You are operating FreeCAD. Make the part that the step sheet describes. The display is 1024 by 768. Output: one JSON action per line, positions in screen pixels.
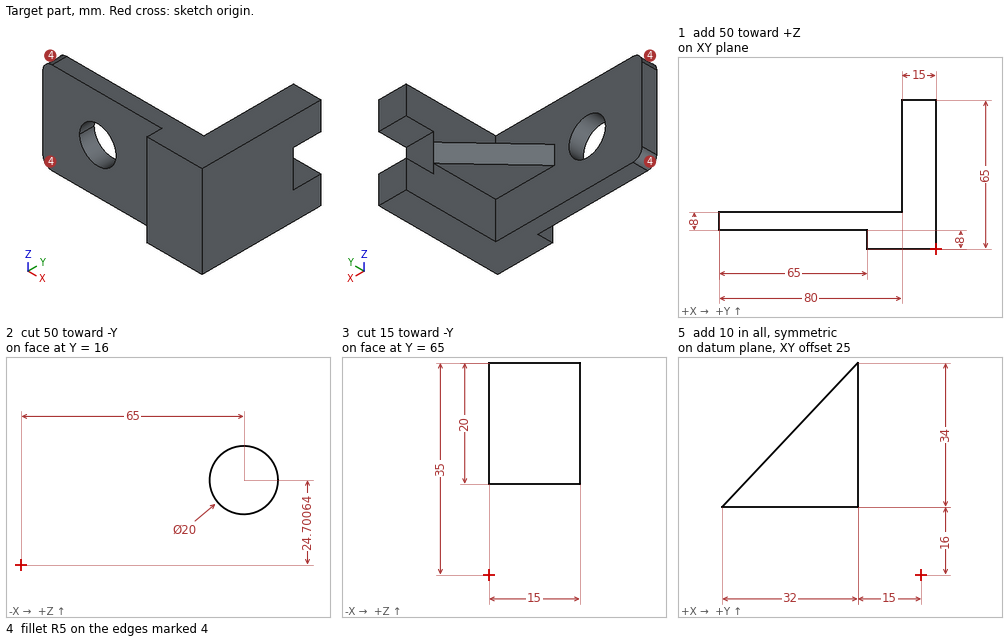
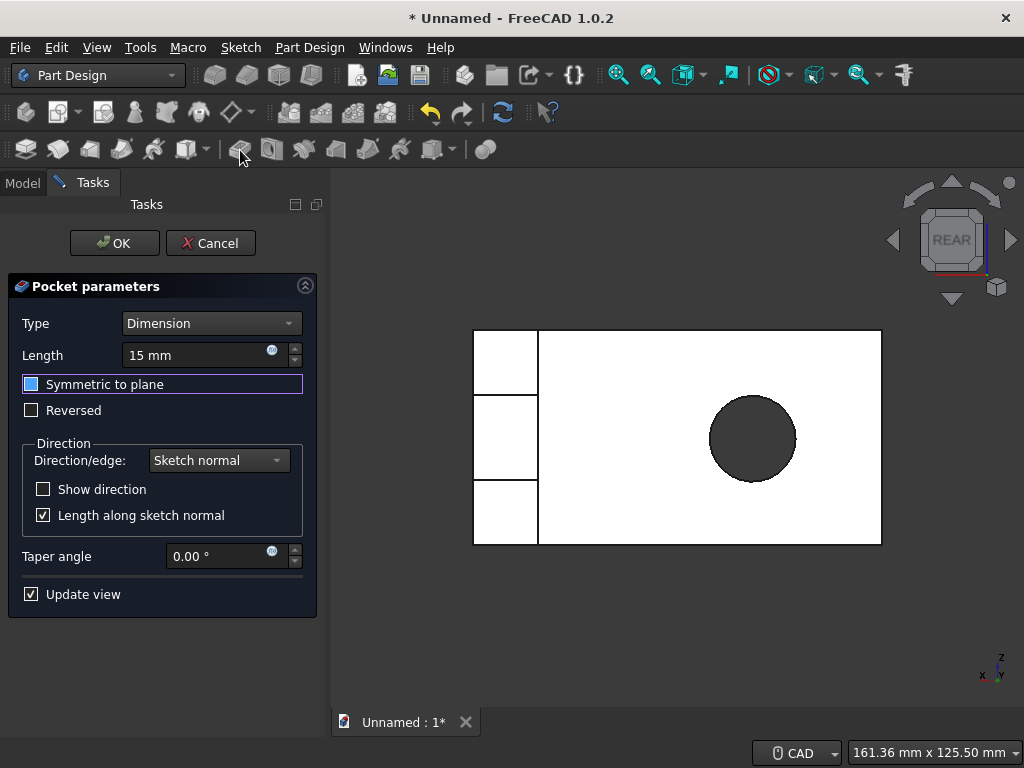
{"action": "left_click", "coordinate": [115, 243]}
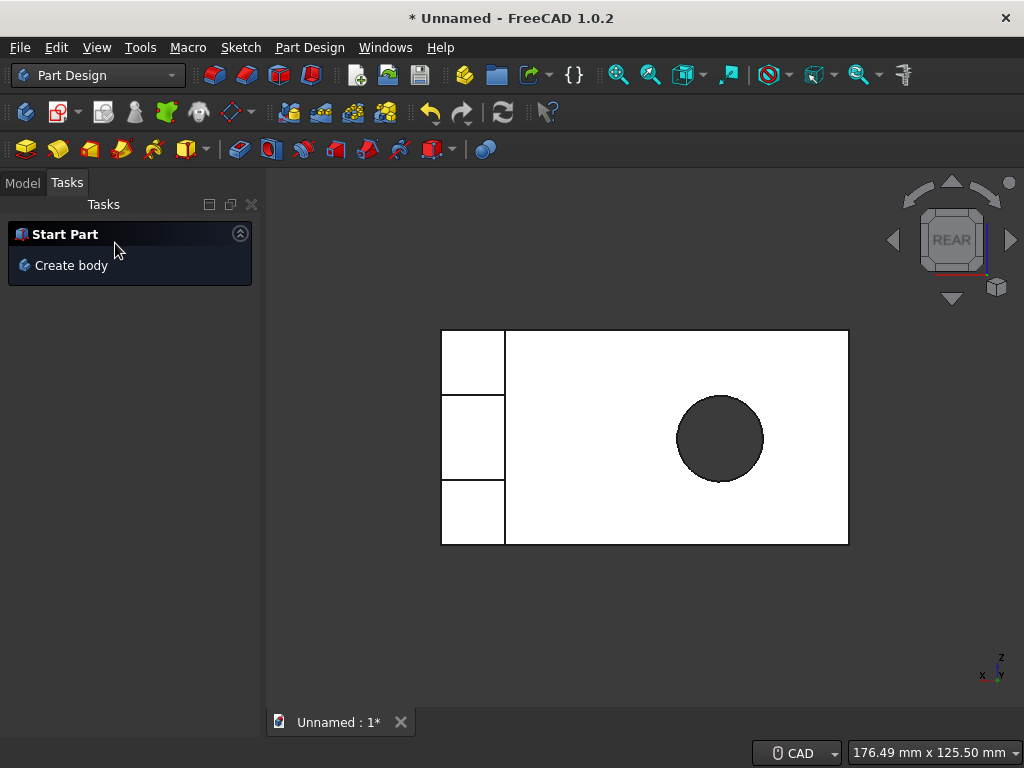
{"action": "key", "text": "0"}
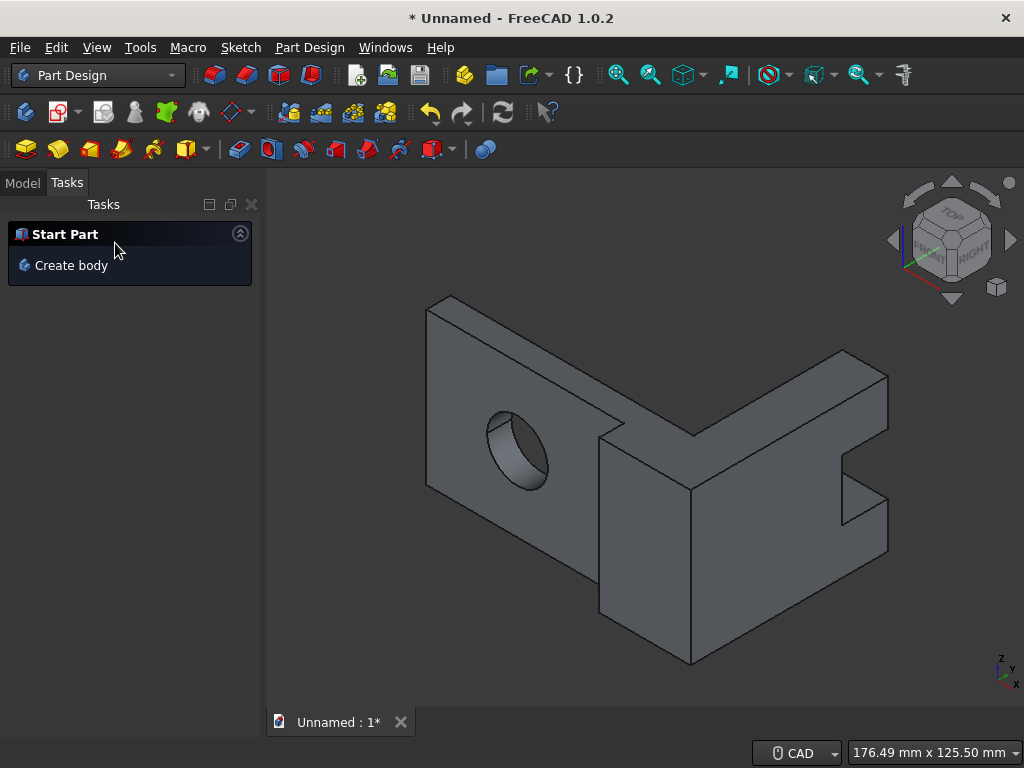
{"action": "key", "text": "2"}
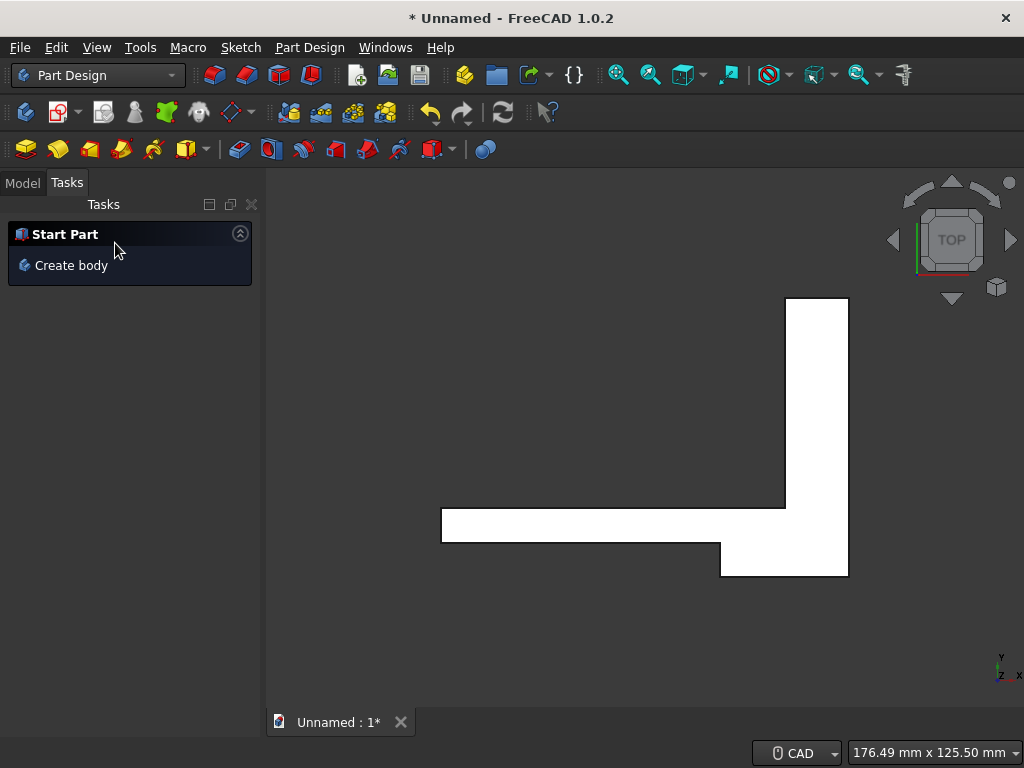
{"action": "left_click", "coordinate": [441, 525]}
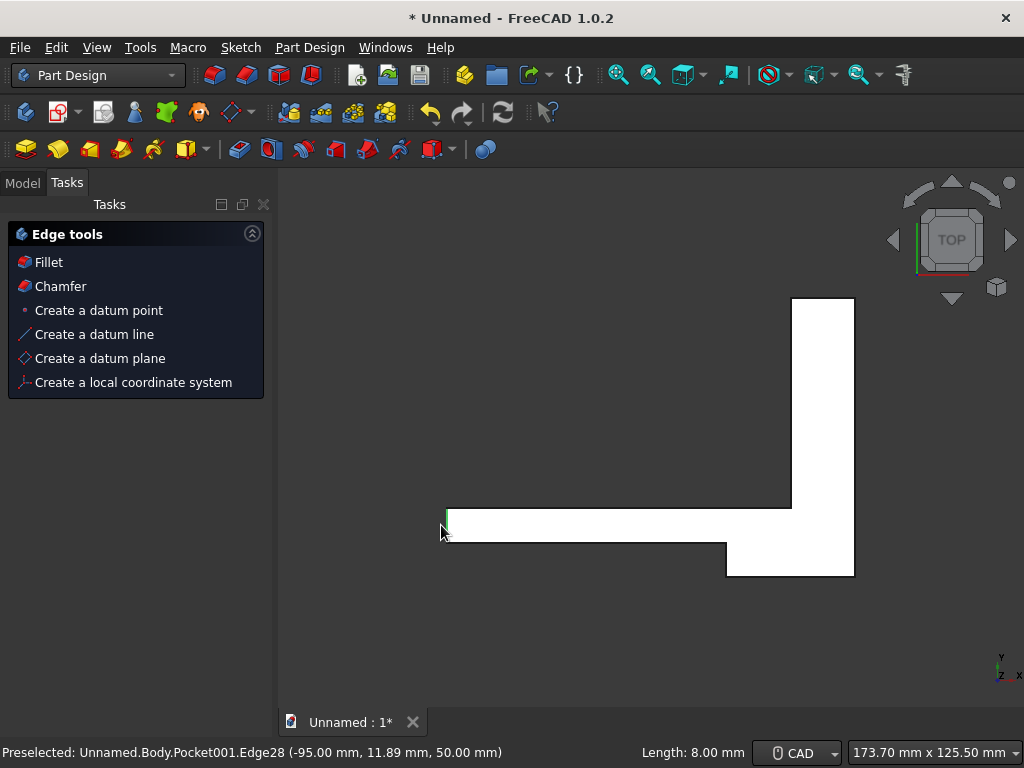
{"action": "key", "text": "1"}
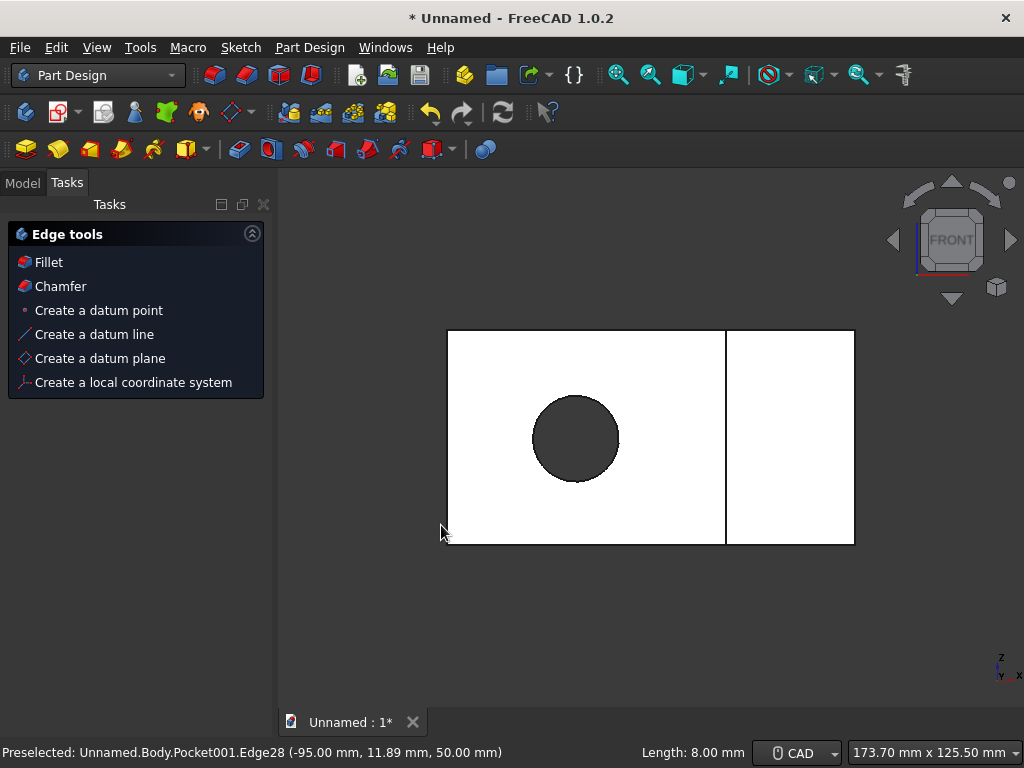
{"action": "key", "text": "3"}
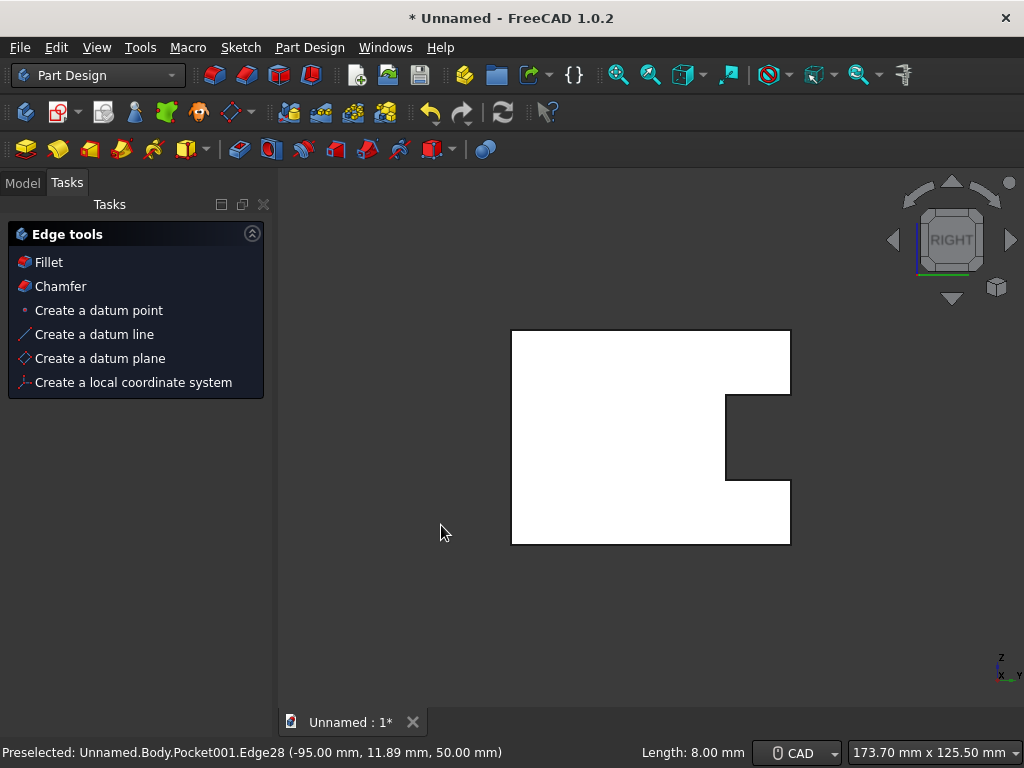
{"action": "left_click", "coordinate": [620, 76]}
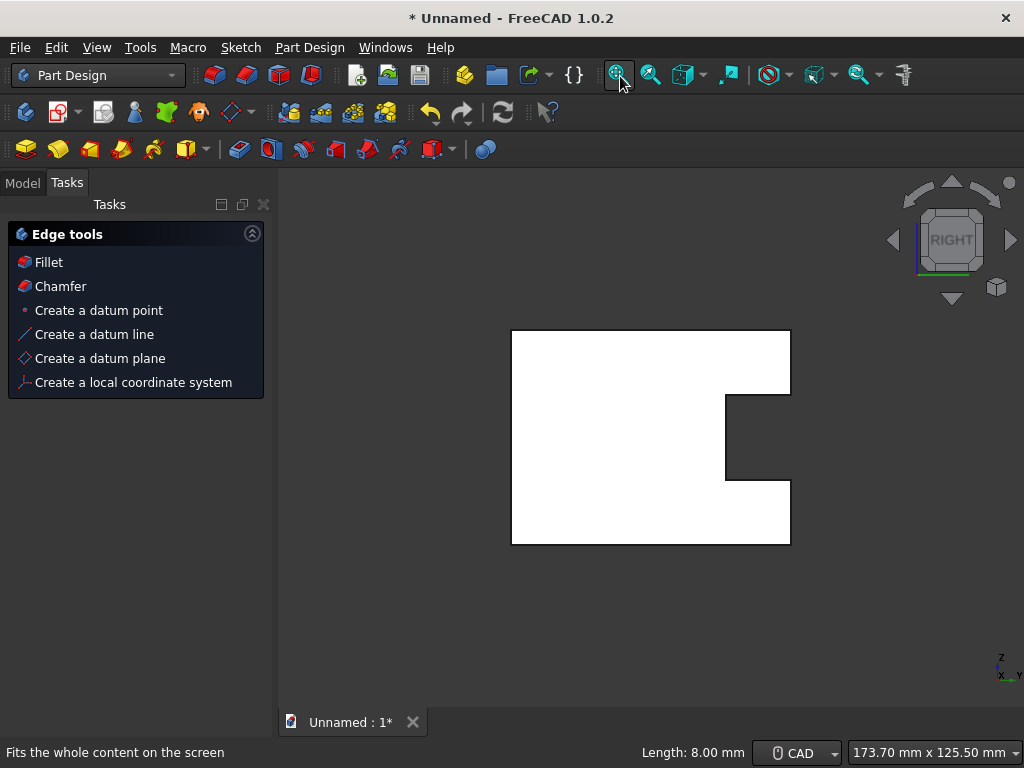
{"action": "key", "text": "5"}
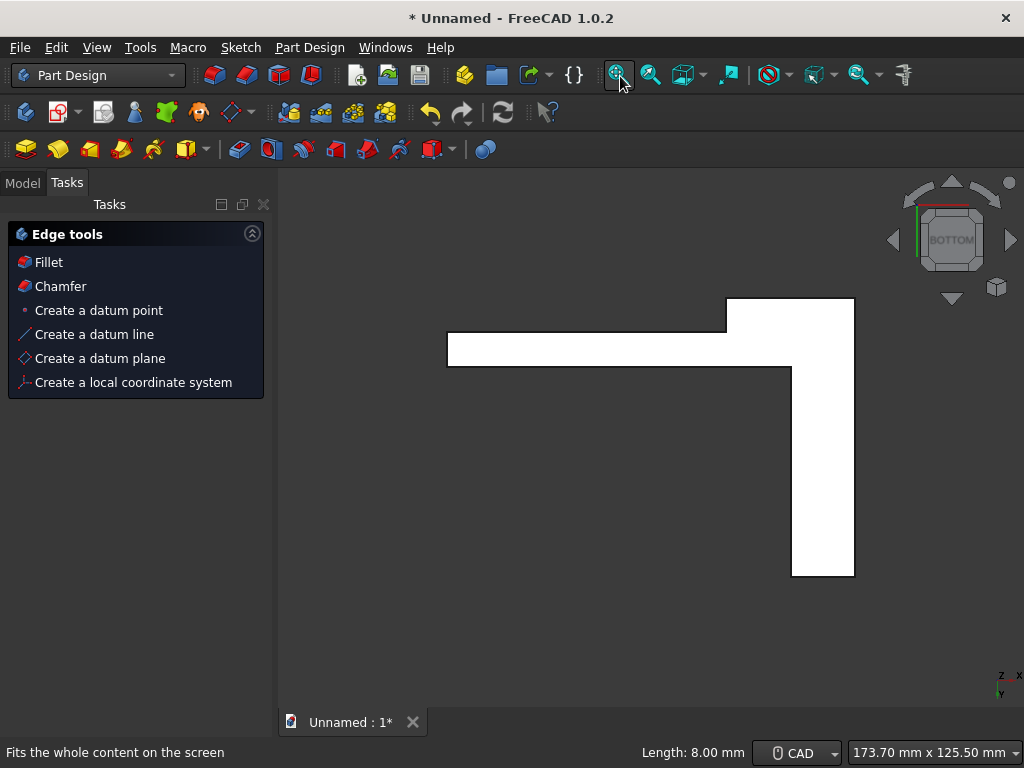
{"action": "left_click", "coordinate": [447, 348], "text": "ctrl"}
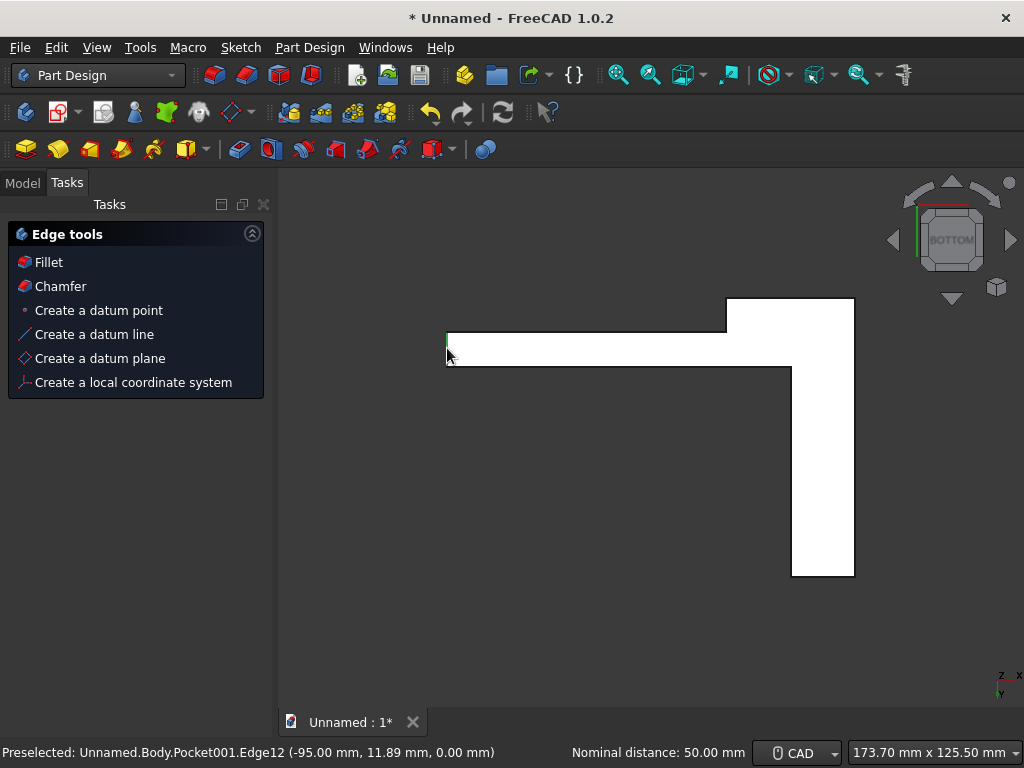
{"action": "left_click", "coordinate": [216, 76]}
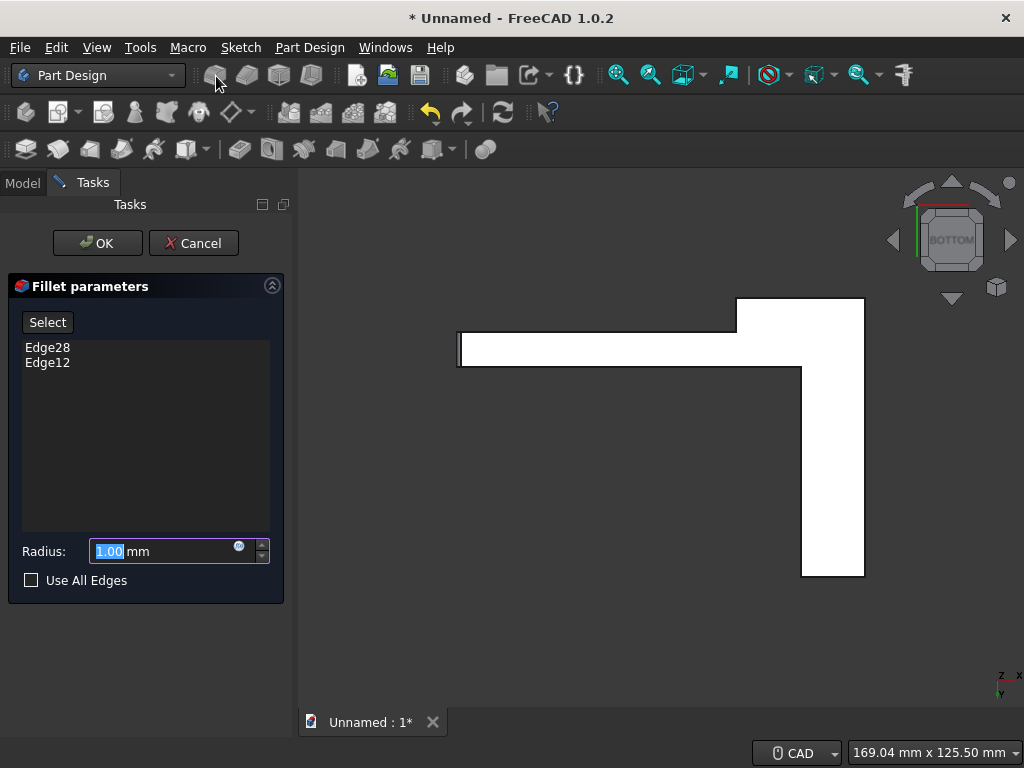
{"action": "type", "text": "5"}
{"action": "key", "text": "Tab"}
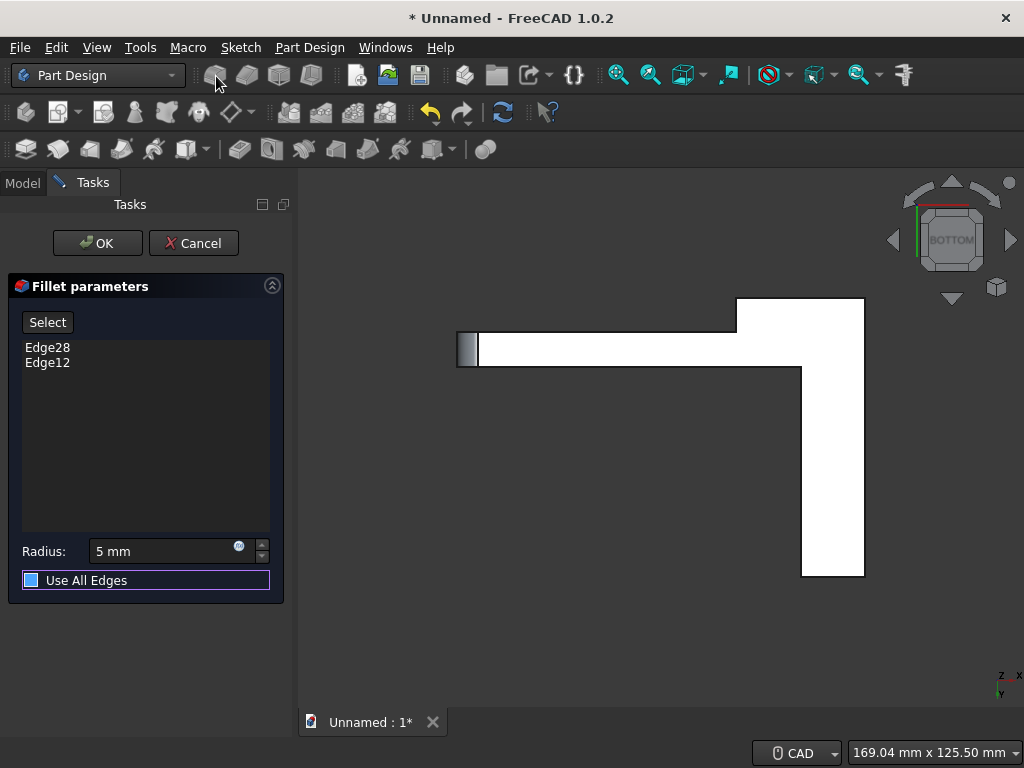
{"action": "left_click", "coordinate": [98, 243]}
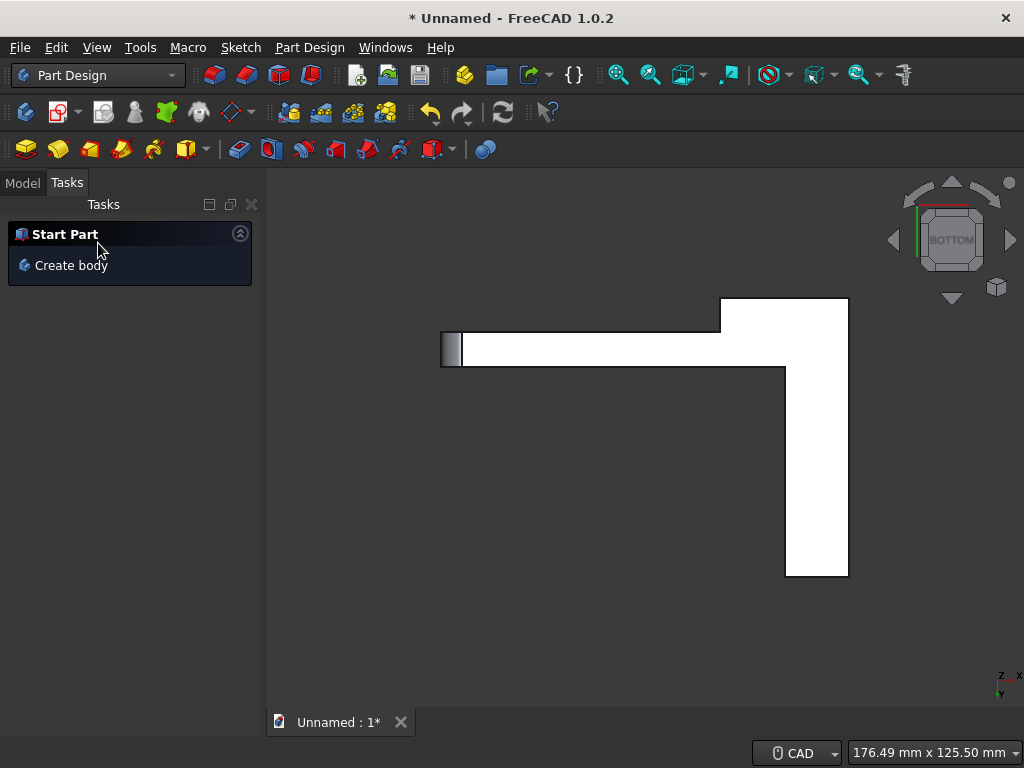
{"action": "left_click", "coordinate": [23, 182]}